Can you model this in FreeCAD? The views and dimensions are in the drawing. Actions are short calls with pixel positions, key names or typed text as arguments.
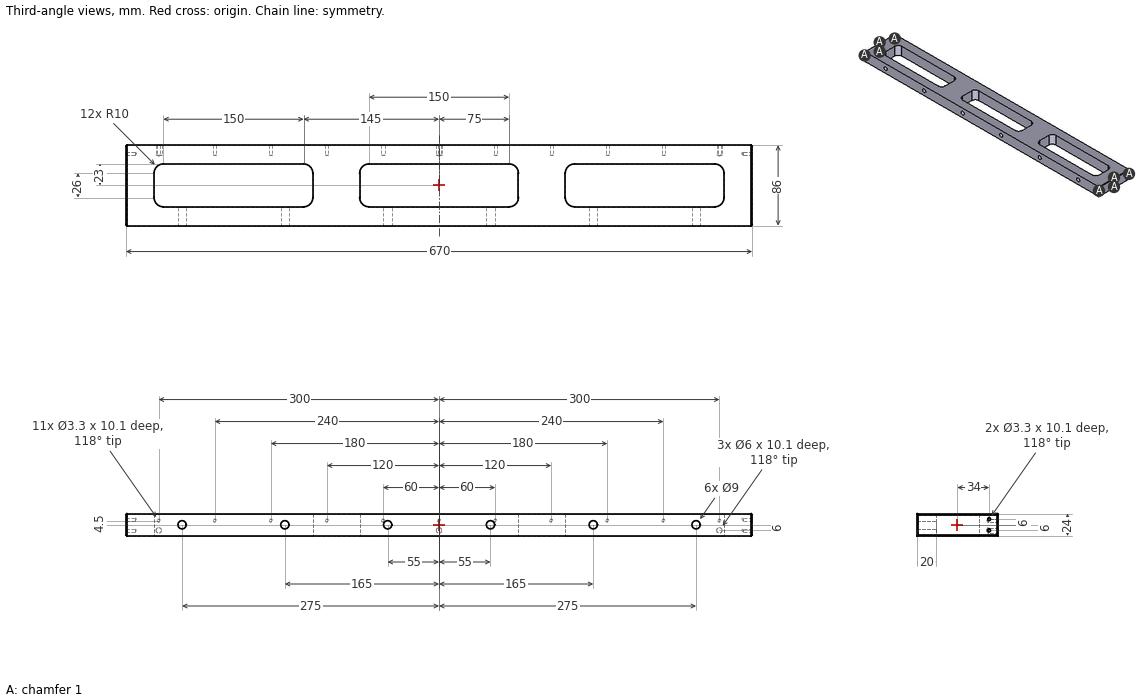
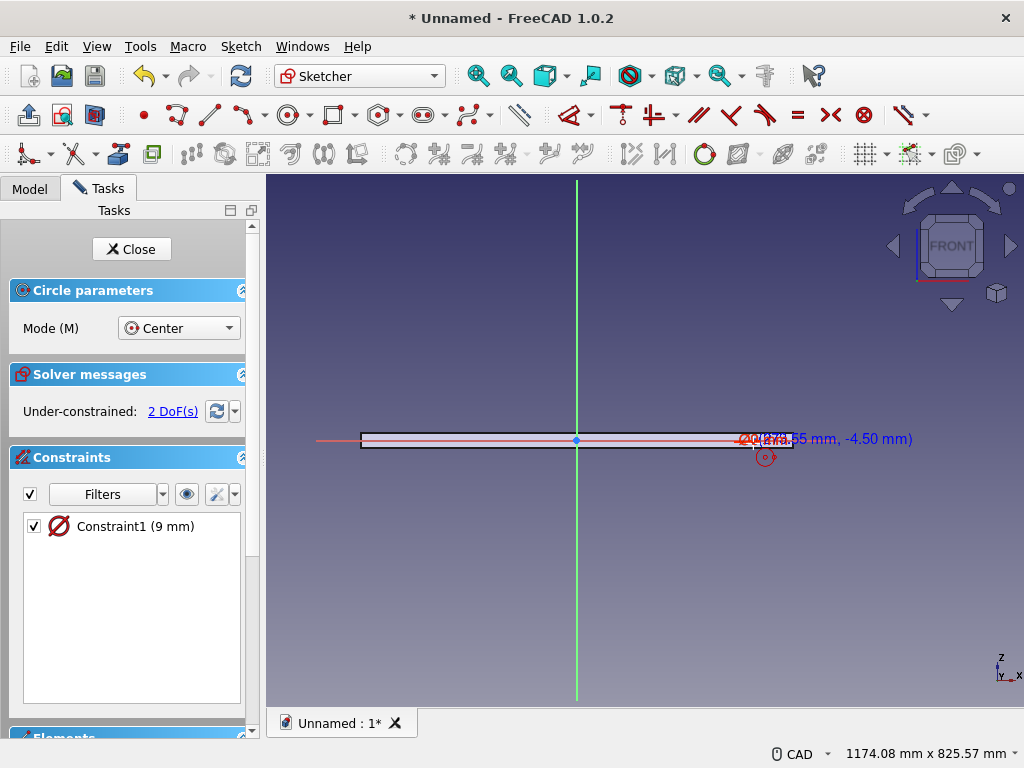
scroll(399, 441, up, 11)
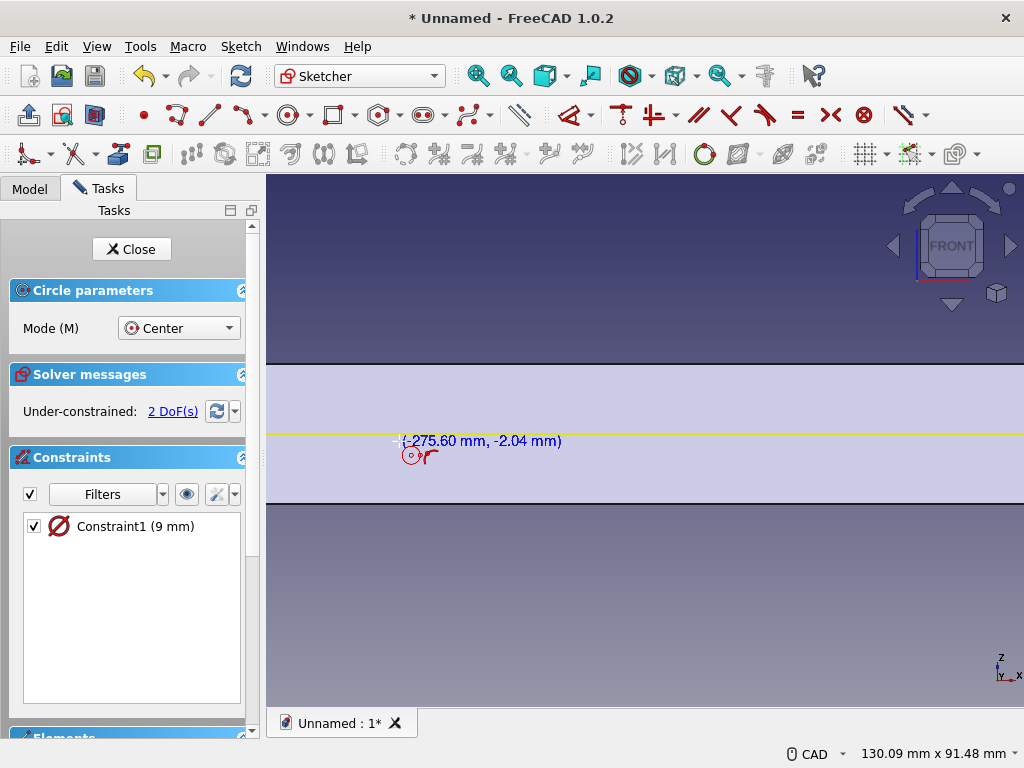
scroll(399, 441, down, 11)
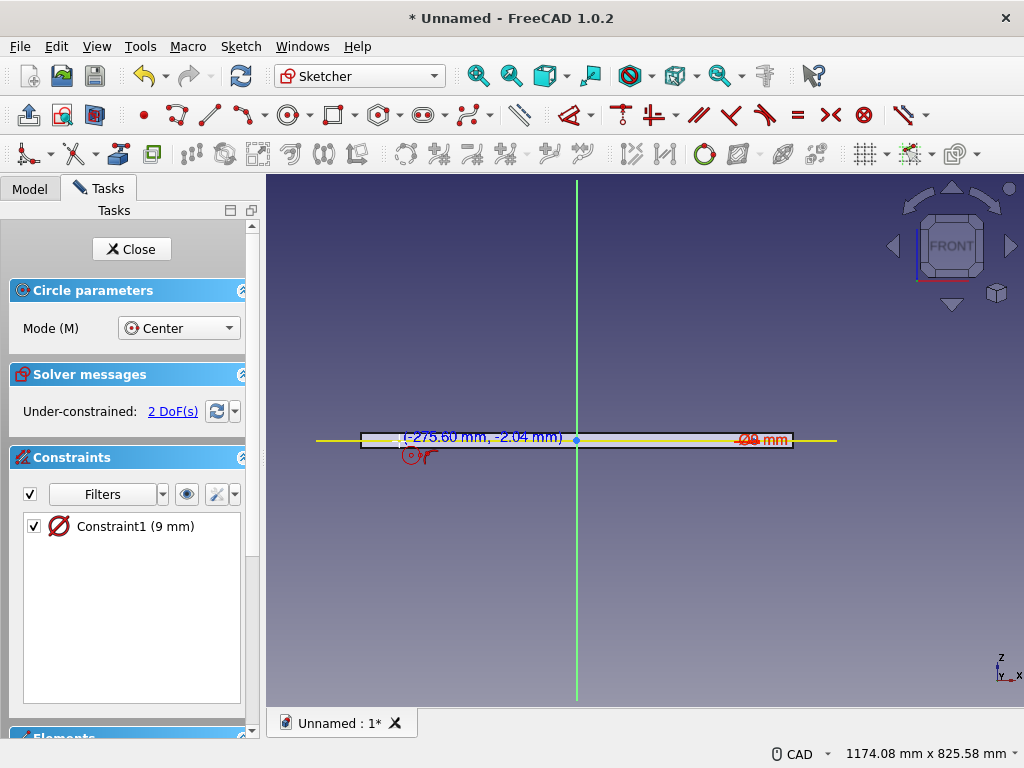
click(399, 441)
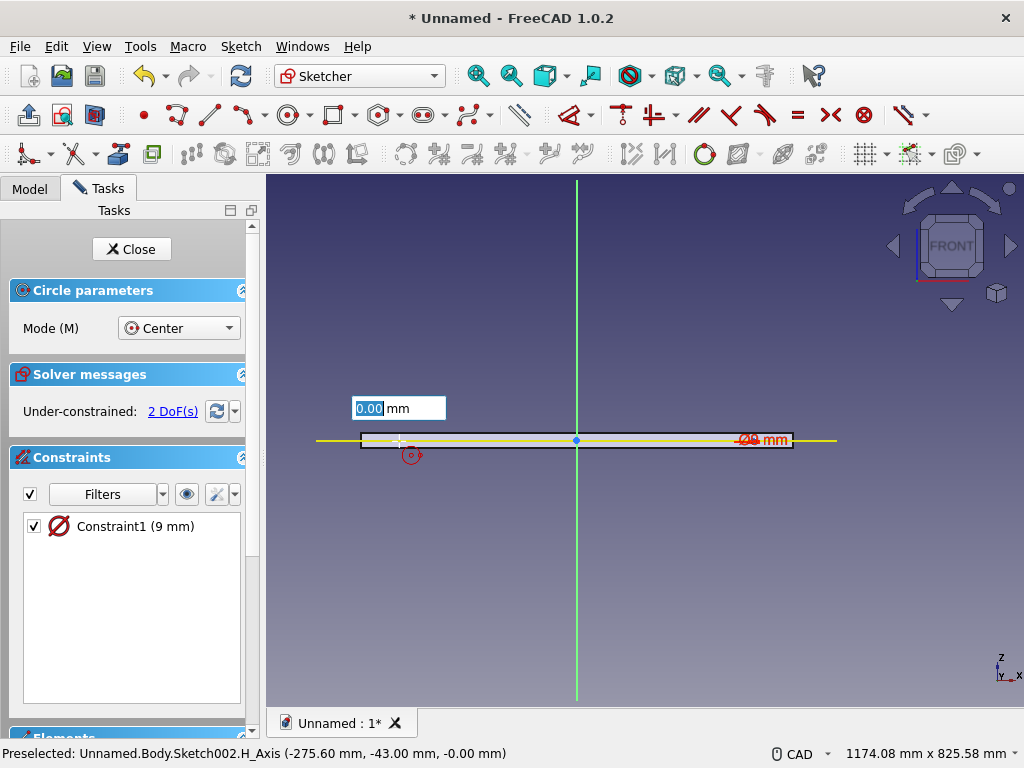
scroll(398, 443, up, 9)
move(399, 443)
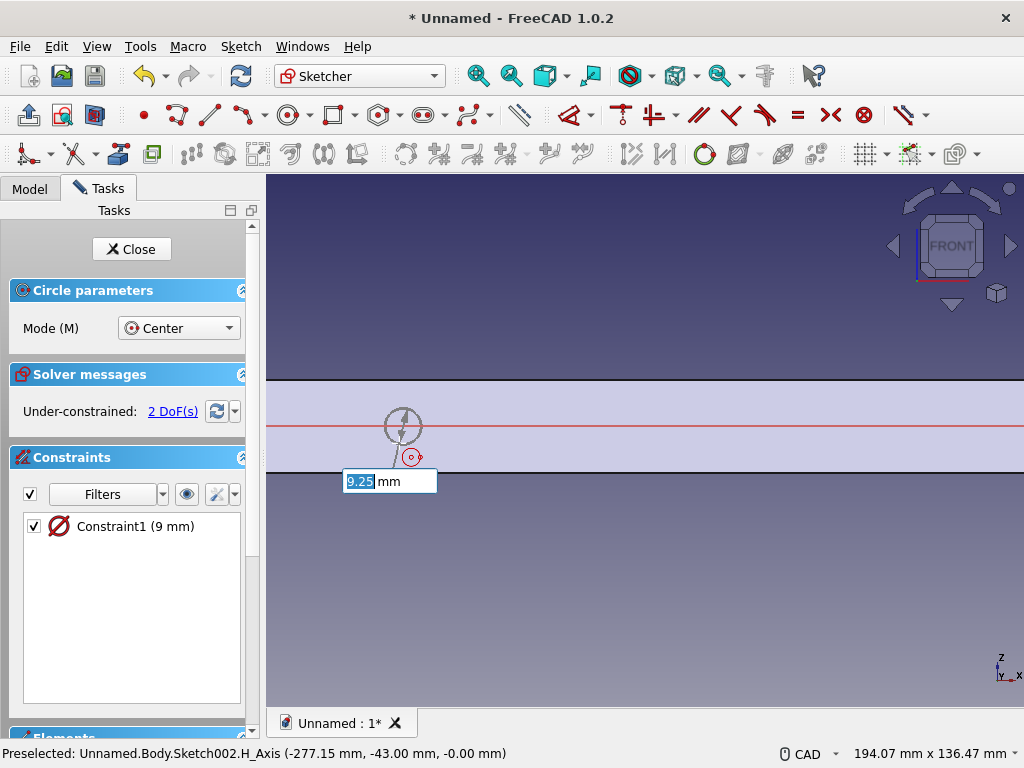
text(9)
key(Return)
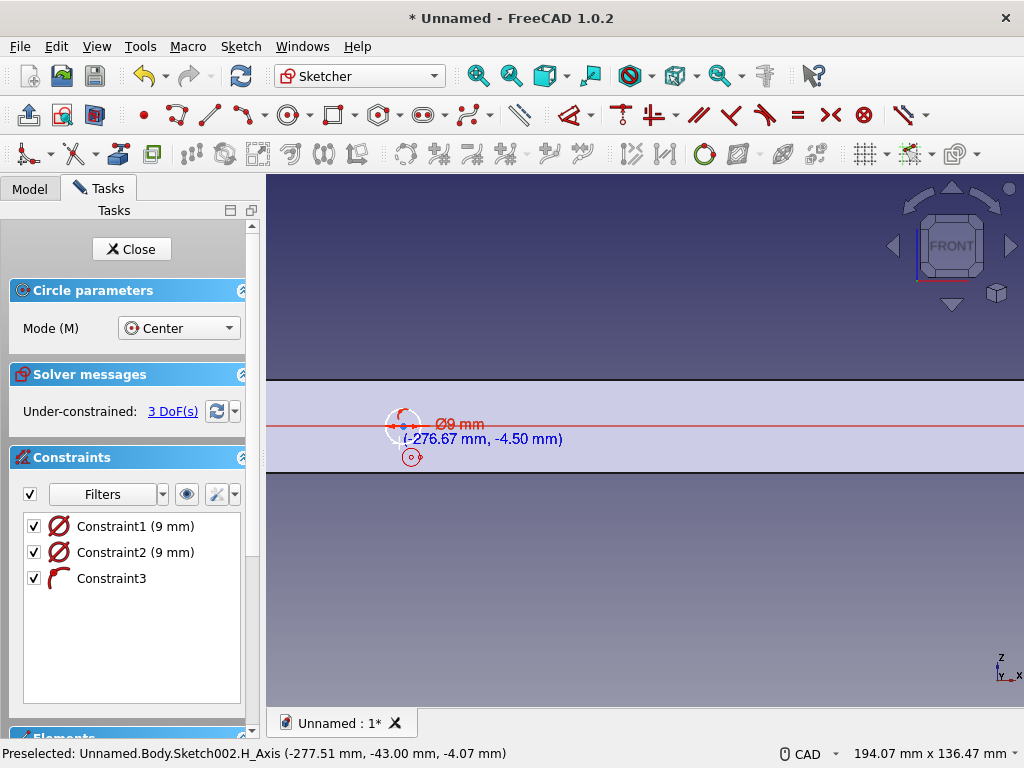
scroll(835, 426, up, 2)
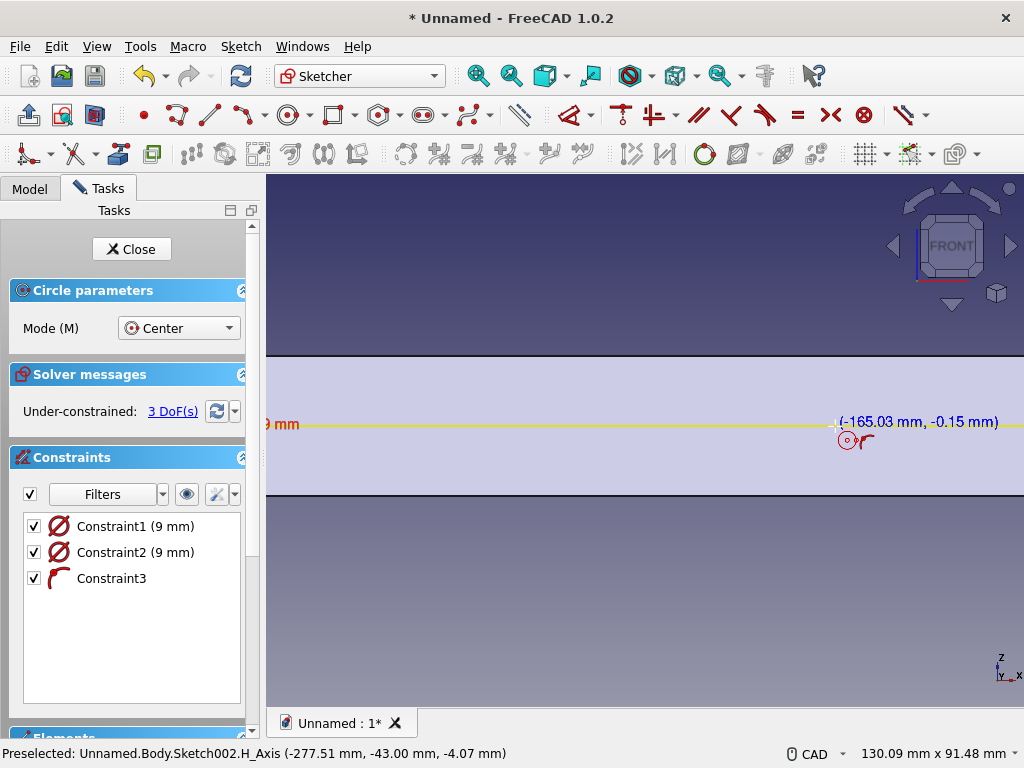
scroll(425, 442, down, 11)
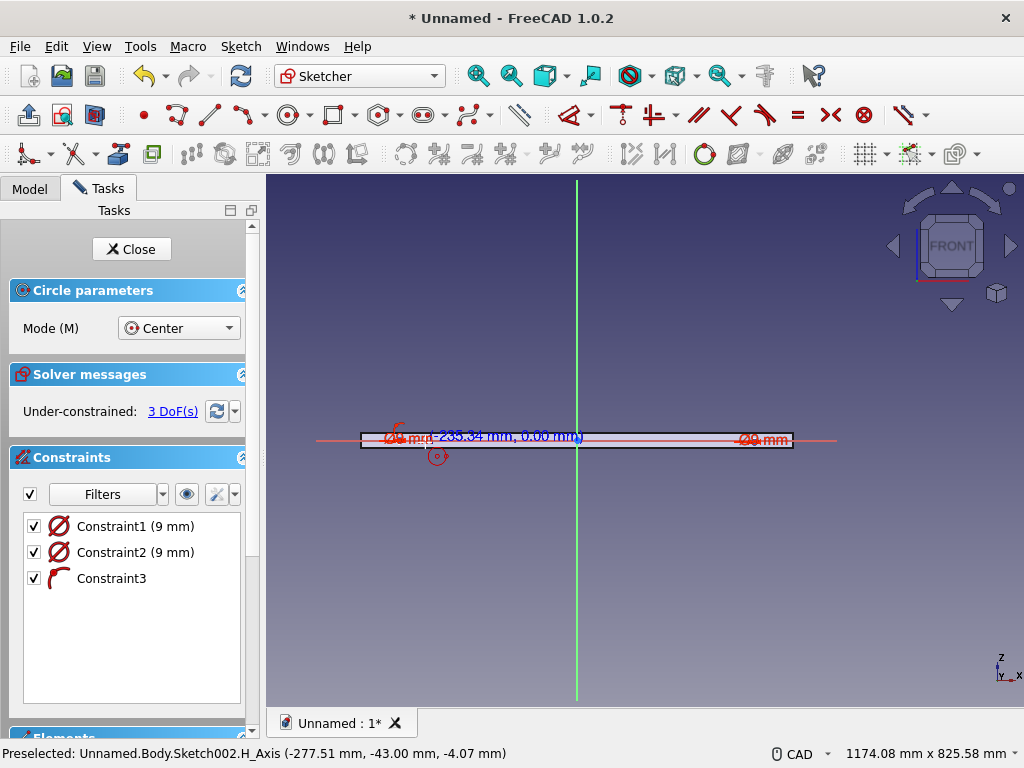
click(471, 441)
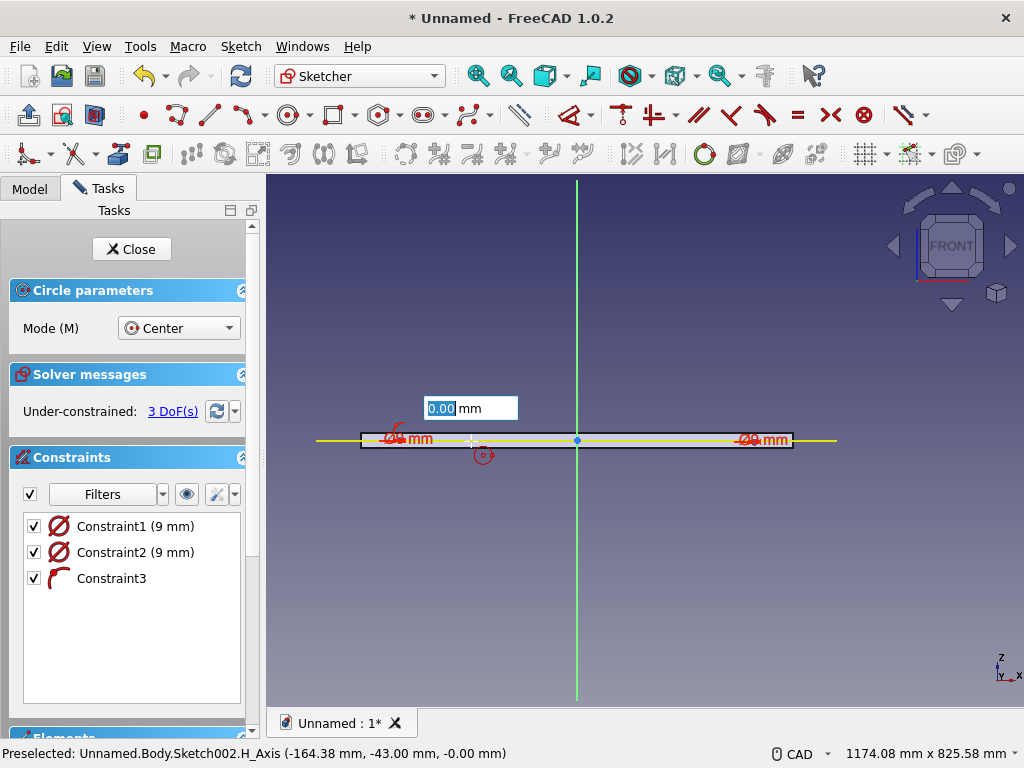
scroll(470, 443, up, 9)
move(466, 443)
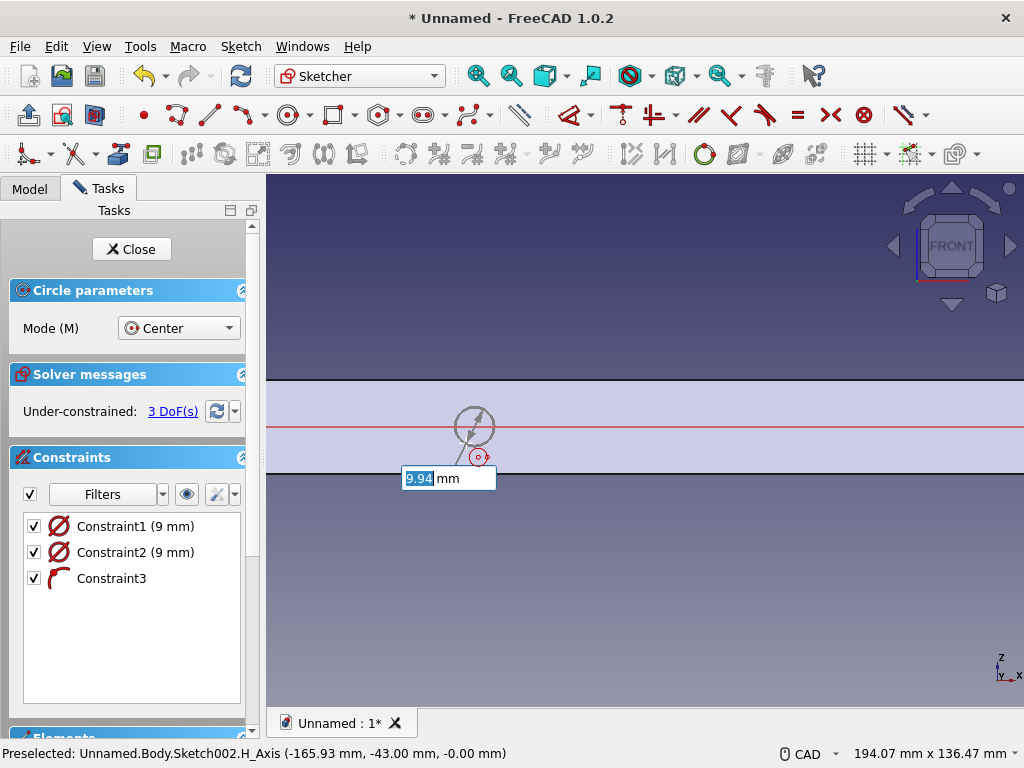
text(9)
key(Return)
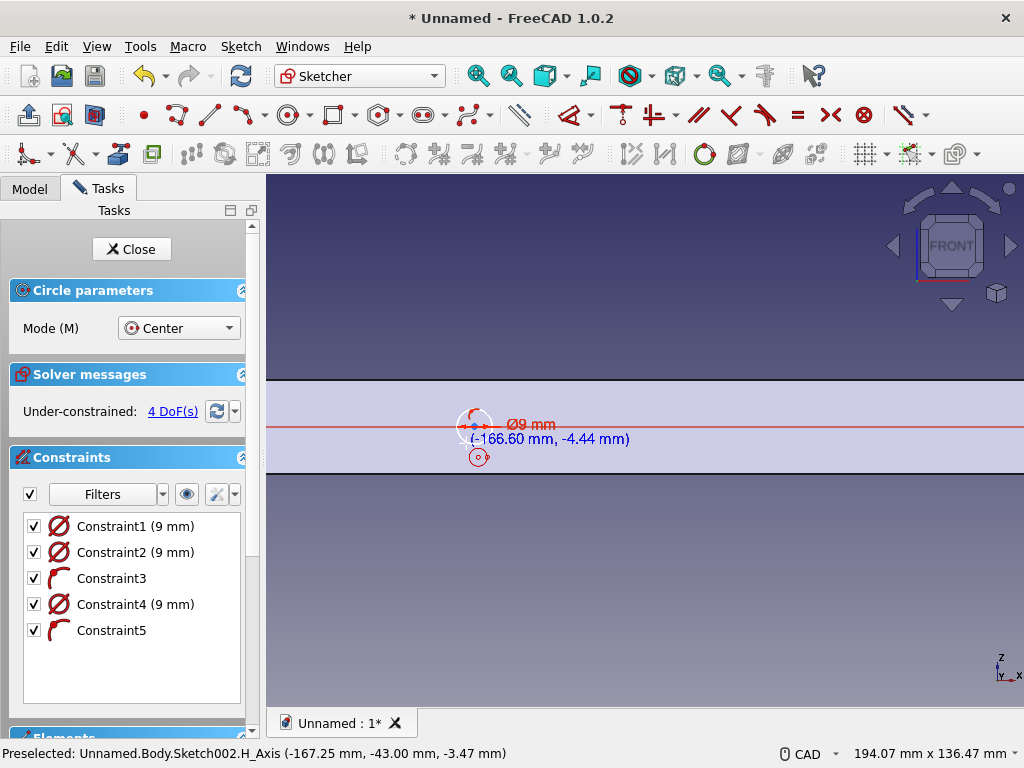
scroll(470, 443, down, 9)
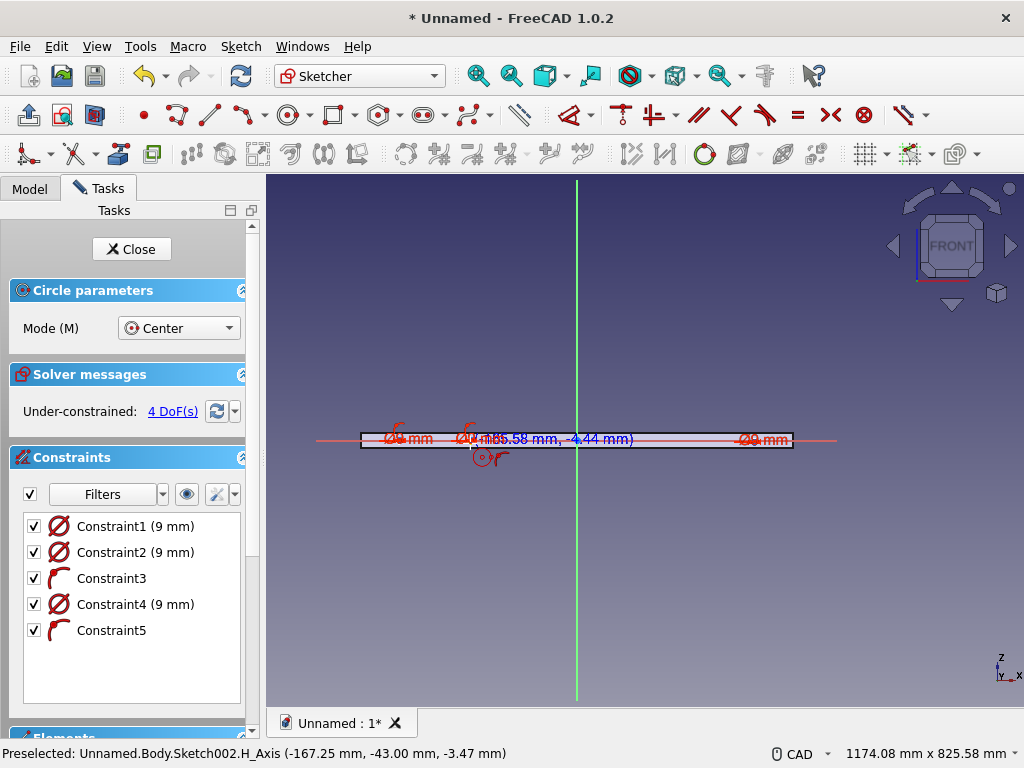
scroll(542, 441, up, 11)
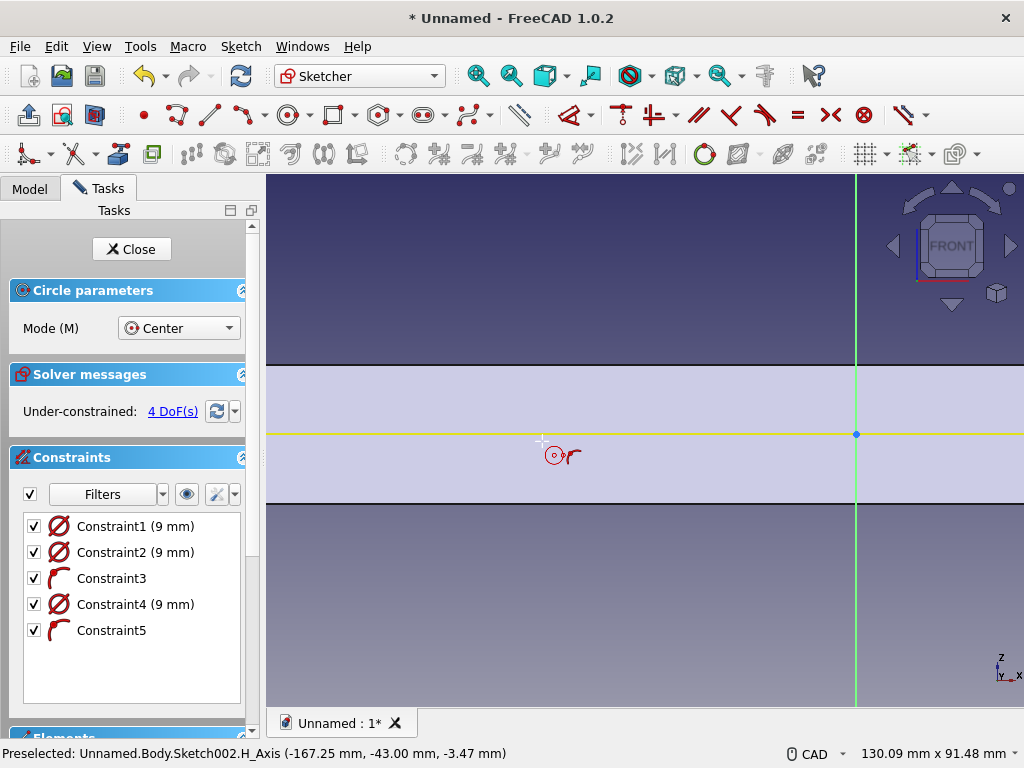
scroll(542, 441, down, 11)